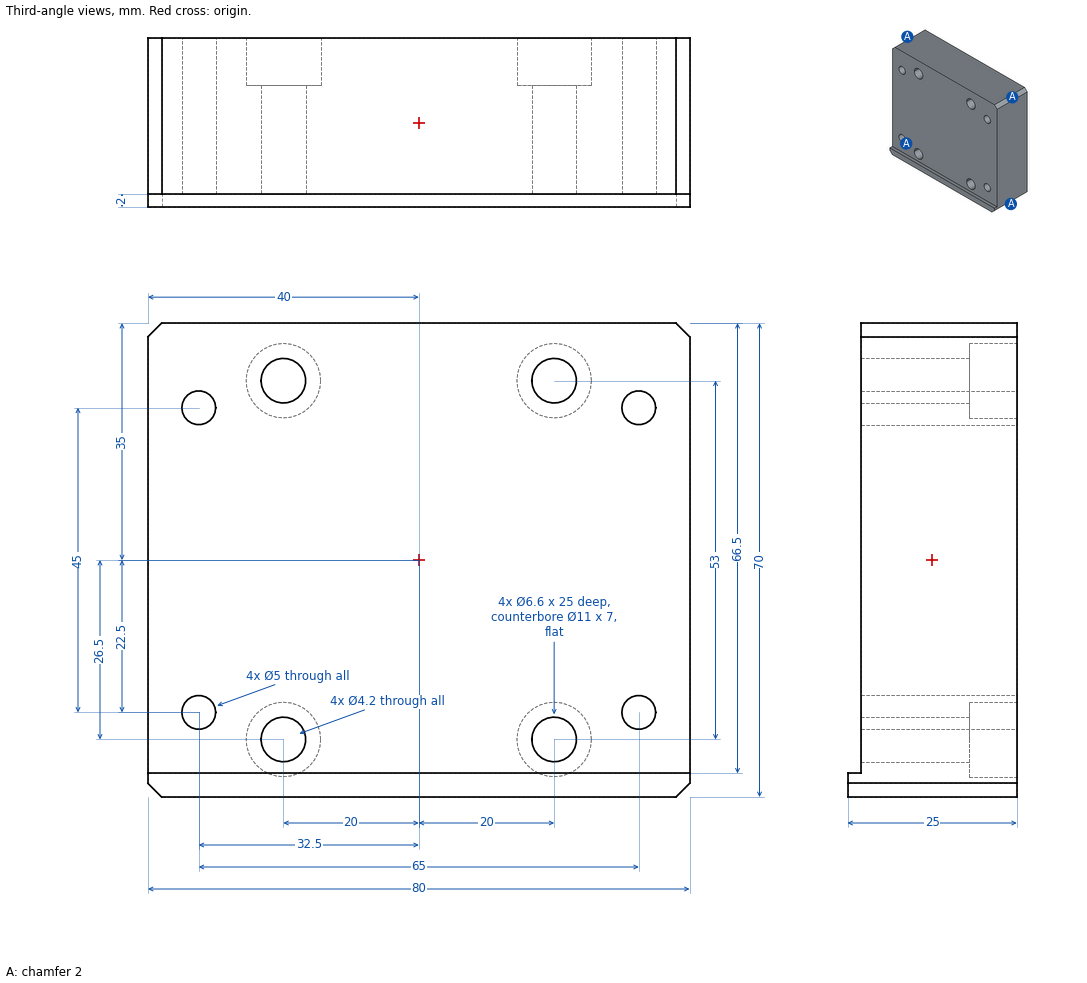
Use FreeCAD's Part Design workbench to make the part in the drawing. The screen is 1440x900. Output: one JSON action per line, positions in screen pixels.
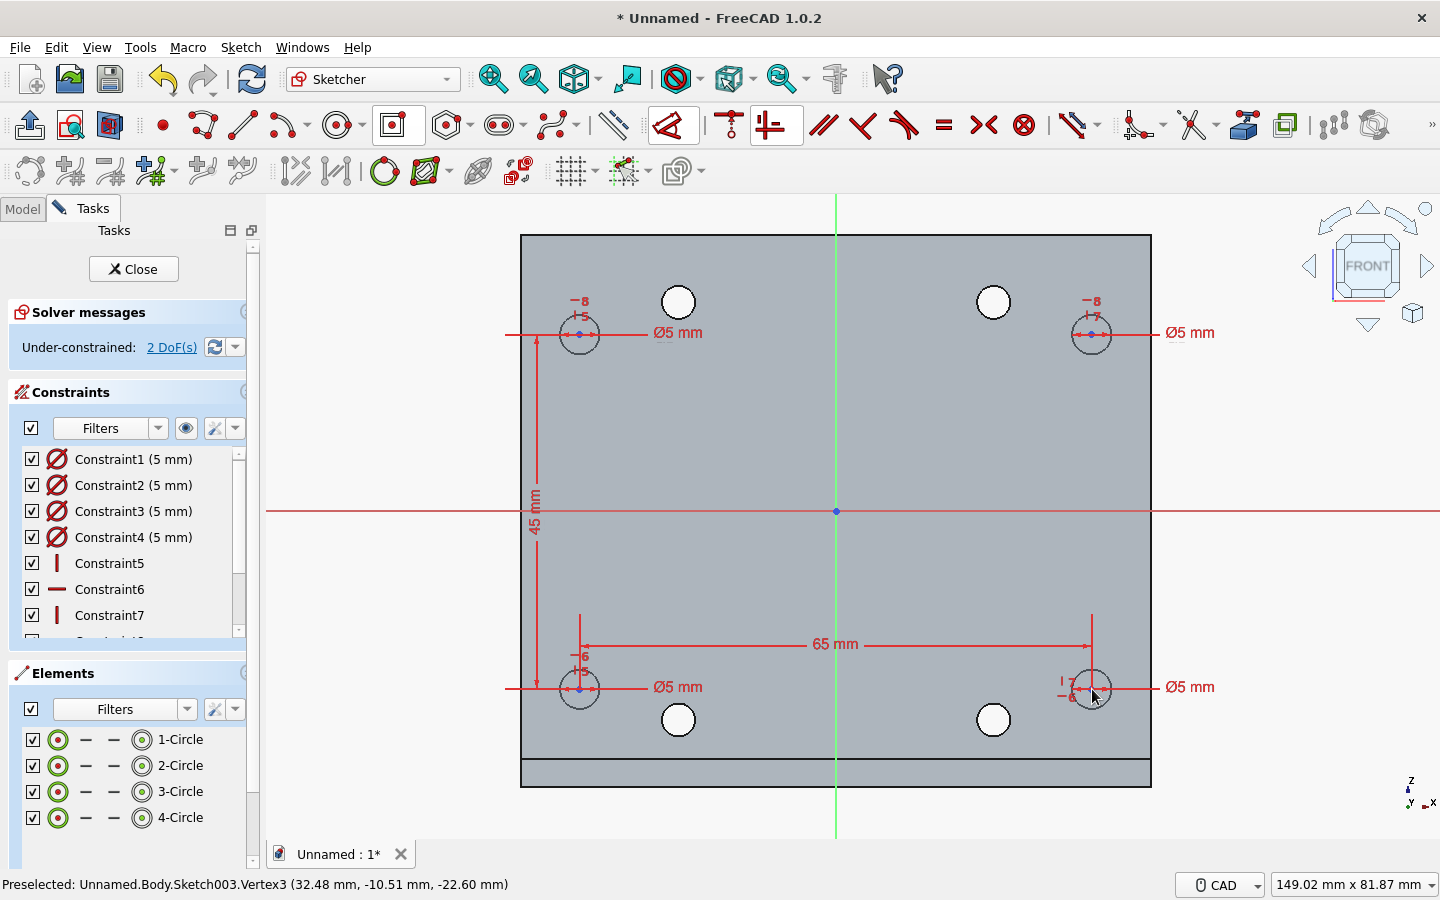
{"action": "left_click", "coordinate": [580, 689]}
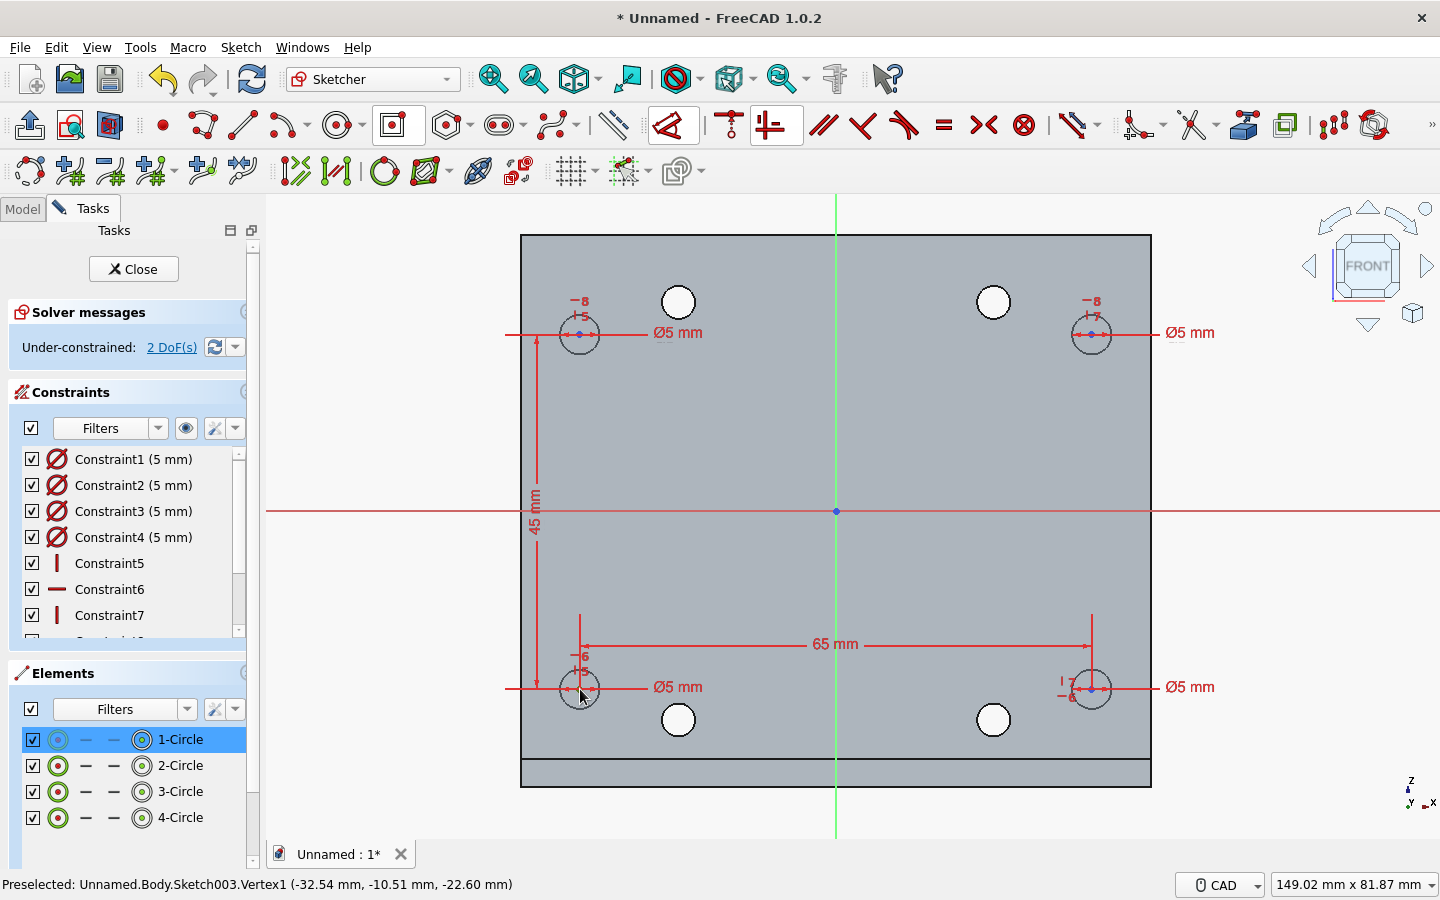
{"action": "left_click", "coordinate": [694, 126]}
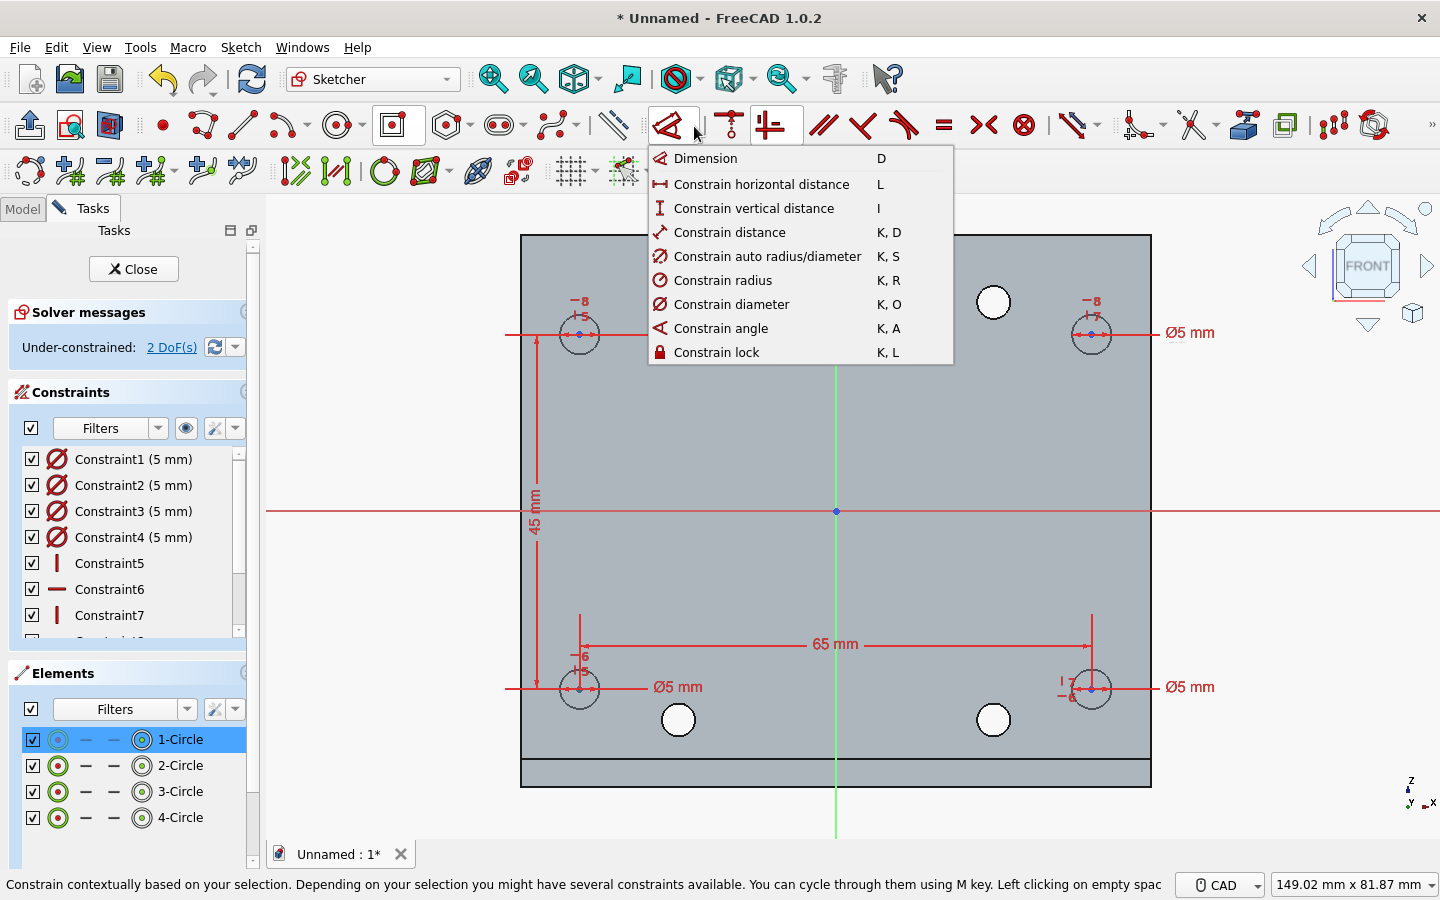
{"action": "left_click", "coordinate": [801, 184]}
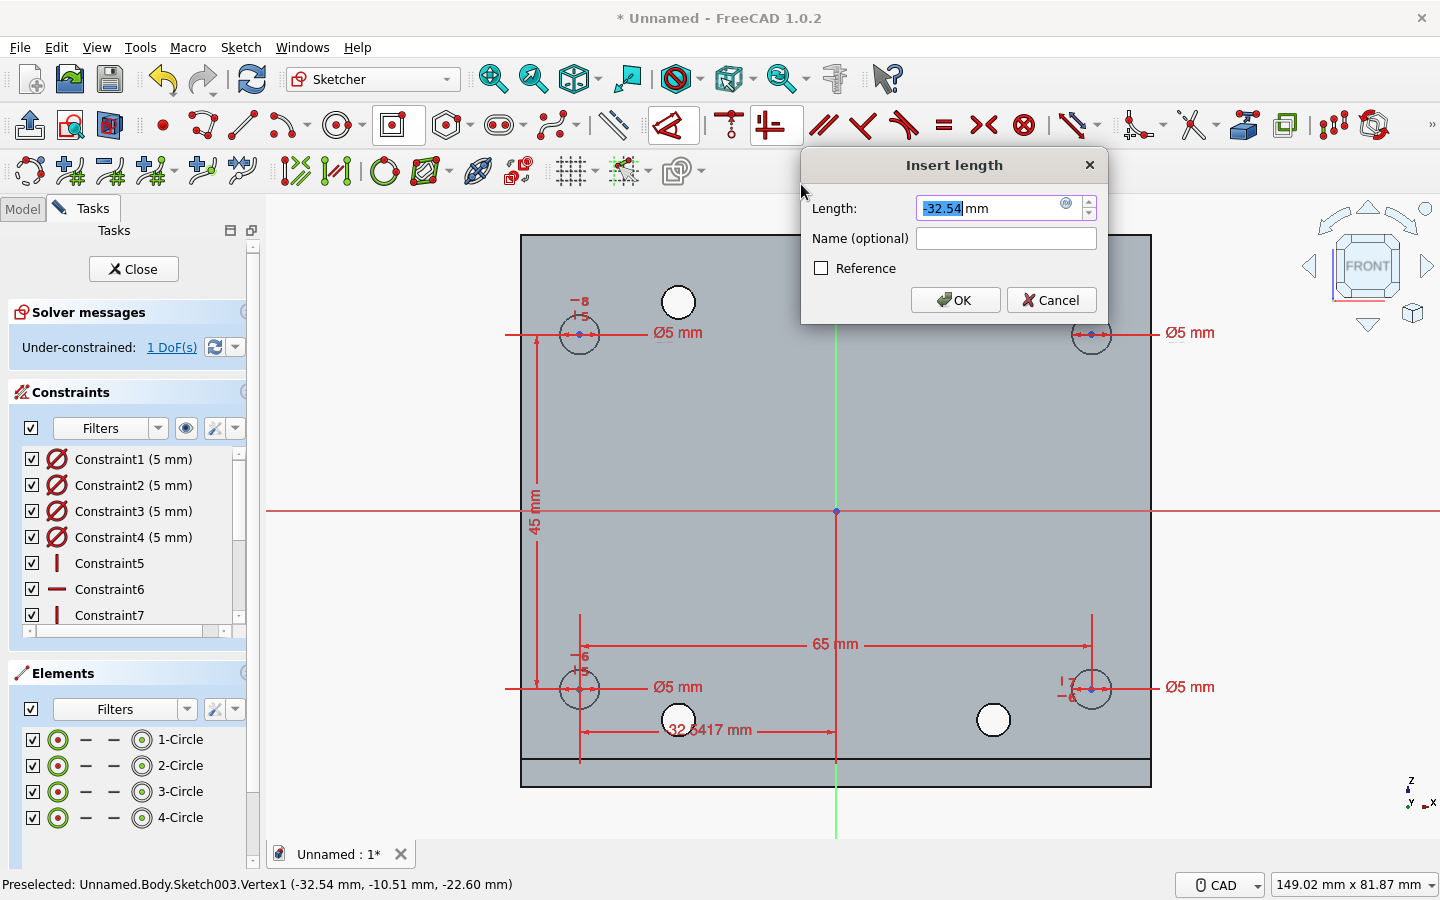
{"action": "type", "text": "-32.5"}
{"action": "key", "text": "Return"}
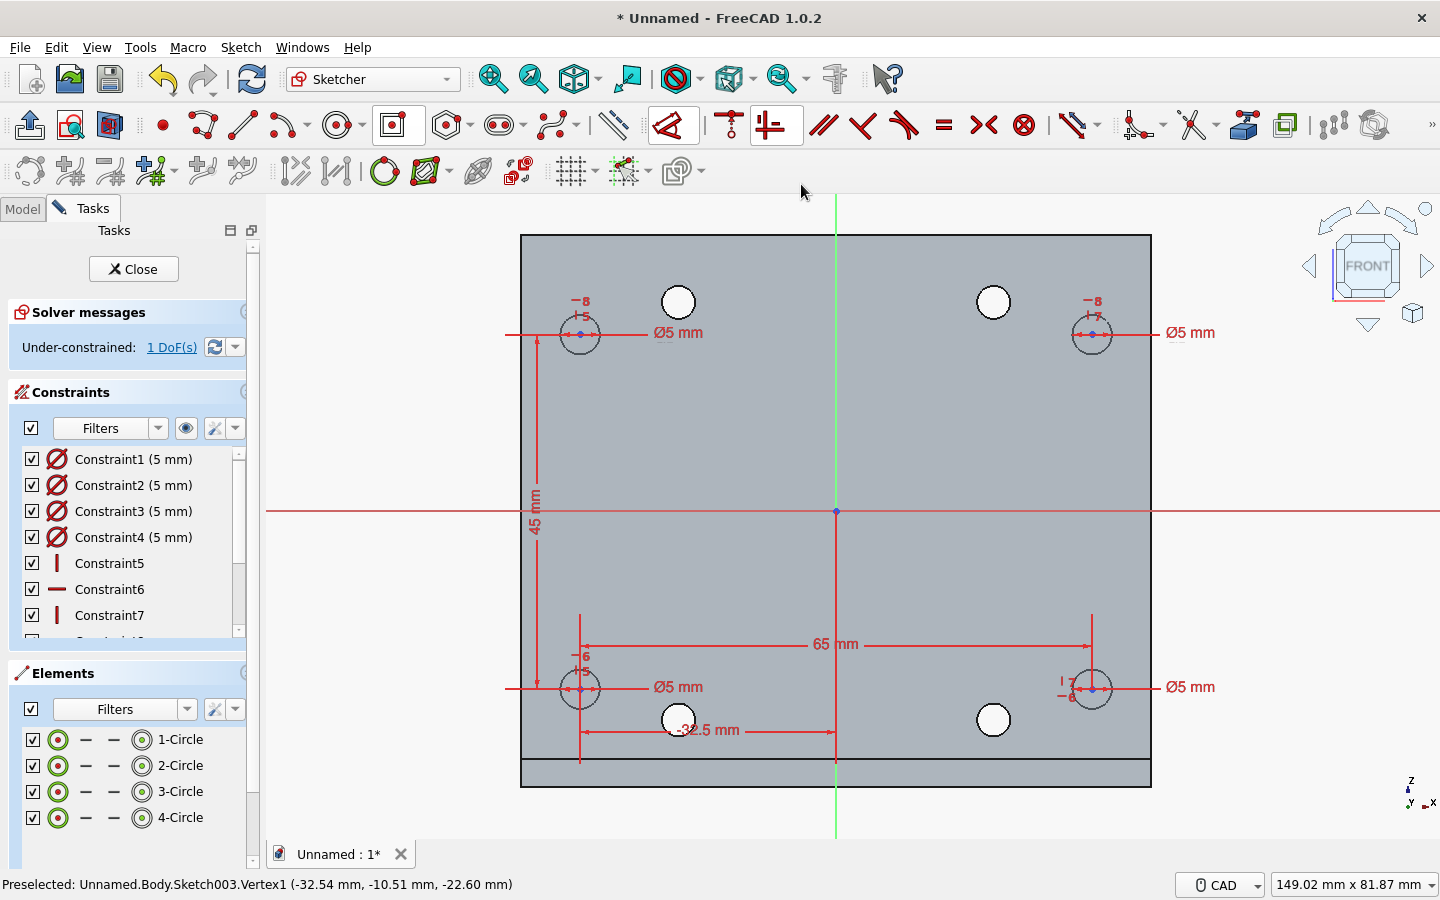
{"action": "left_click", "coordinate": [580, 689]}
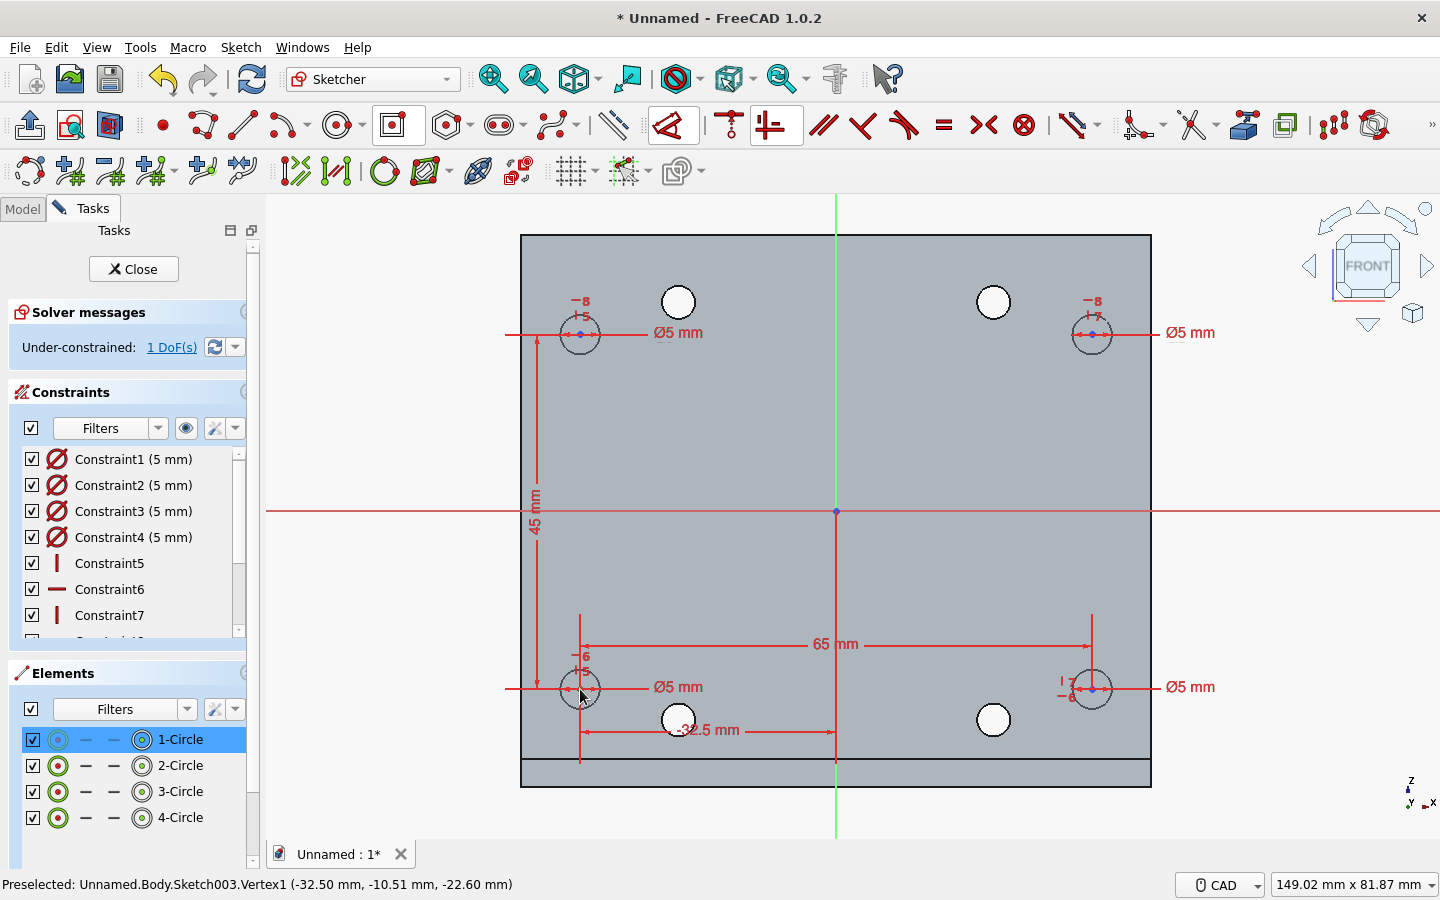
{"action": "left_click", "coordinate": [694, 126]}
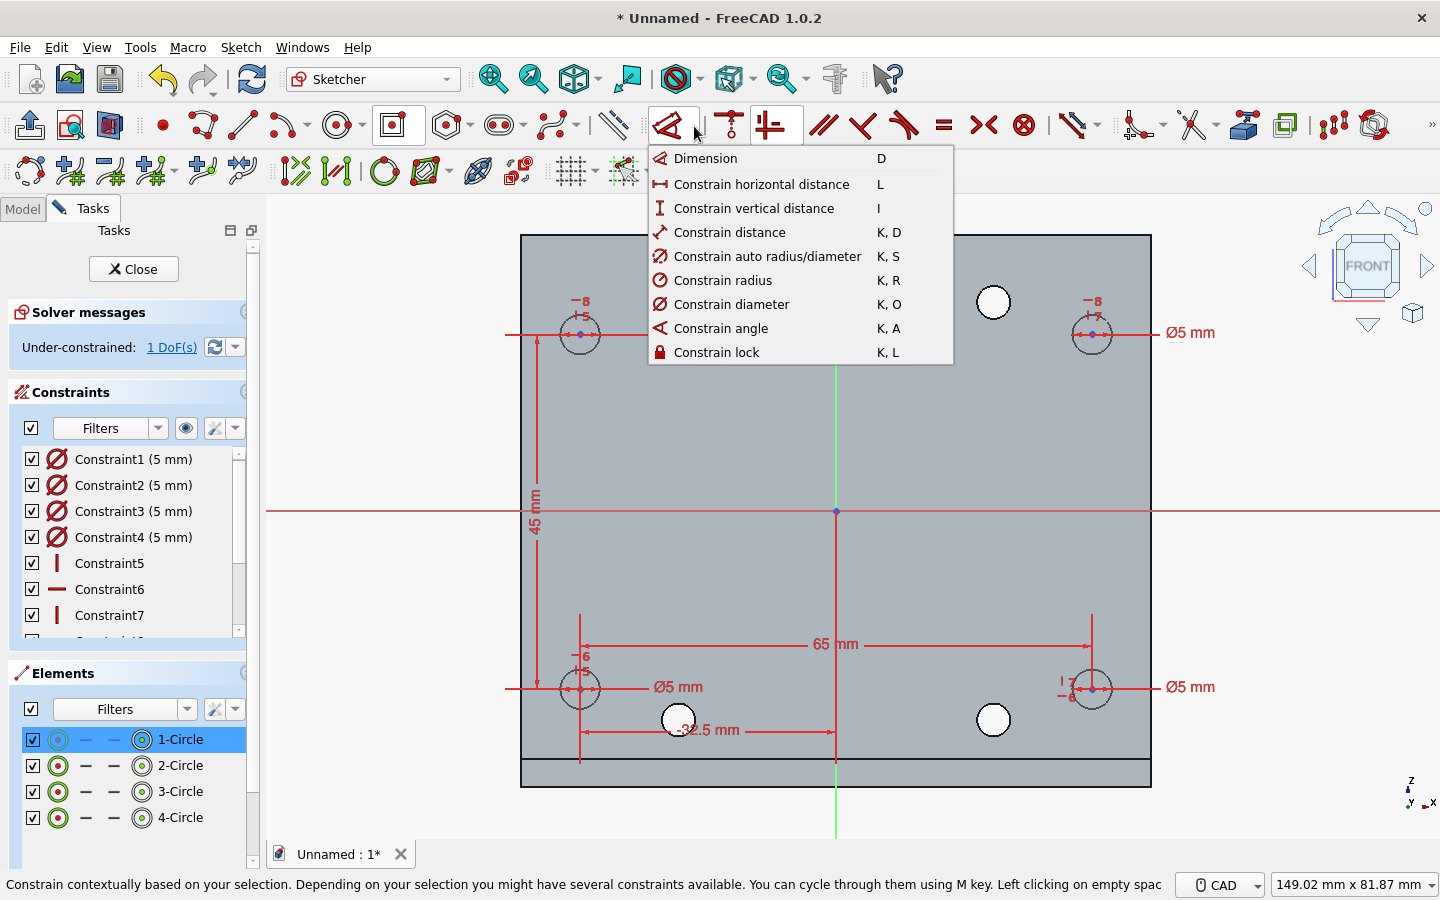
{"action": "left_click", "coordinate": [801, 208]}